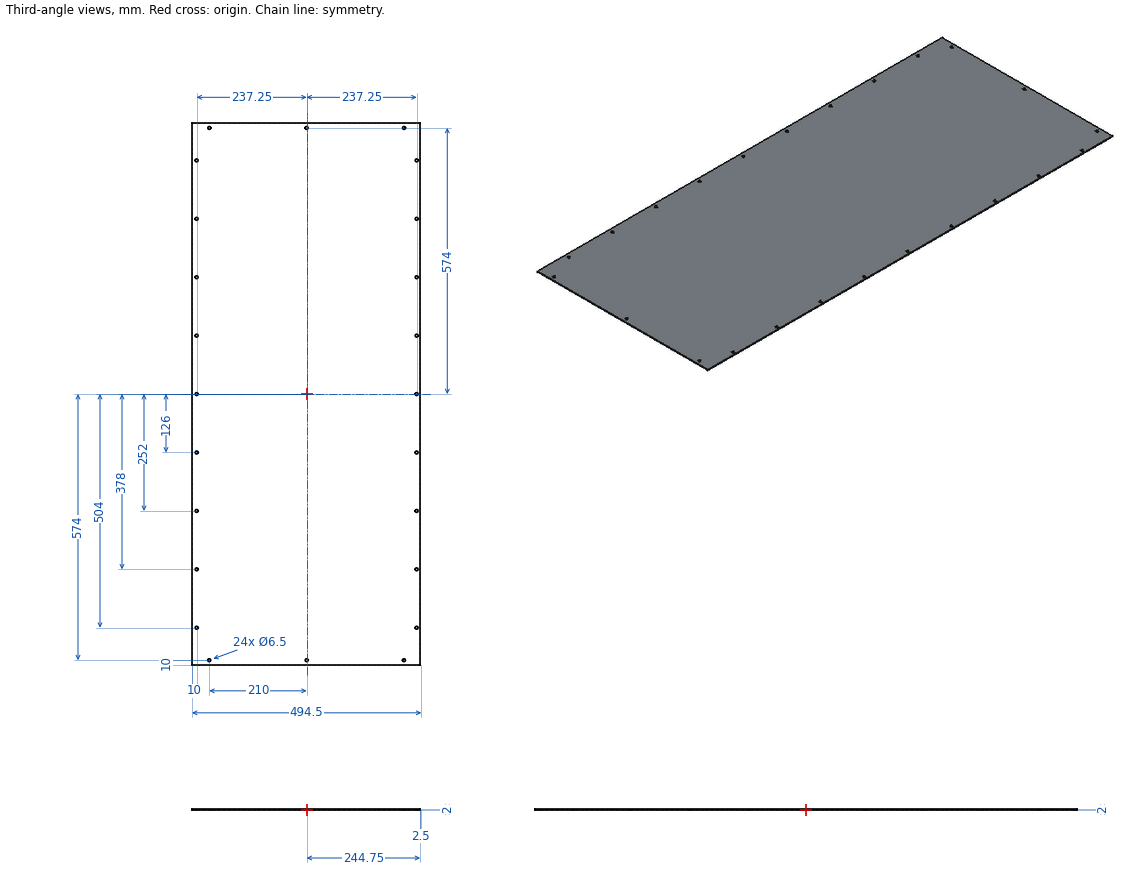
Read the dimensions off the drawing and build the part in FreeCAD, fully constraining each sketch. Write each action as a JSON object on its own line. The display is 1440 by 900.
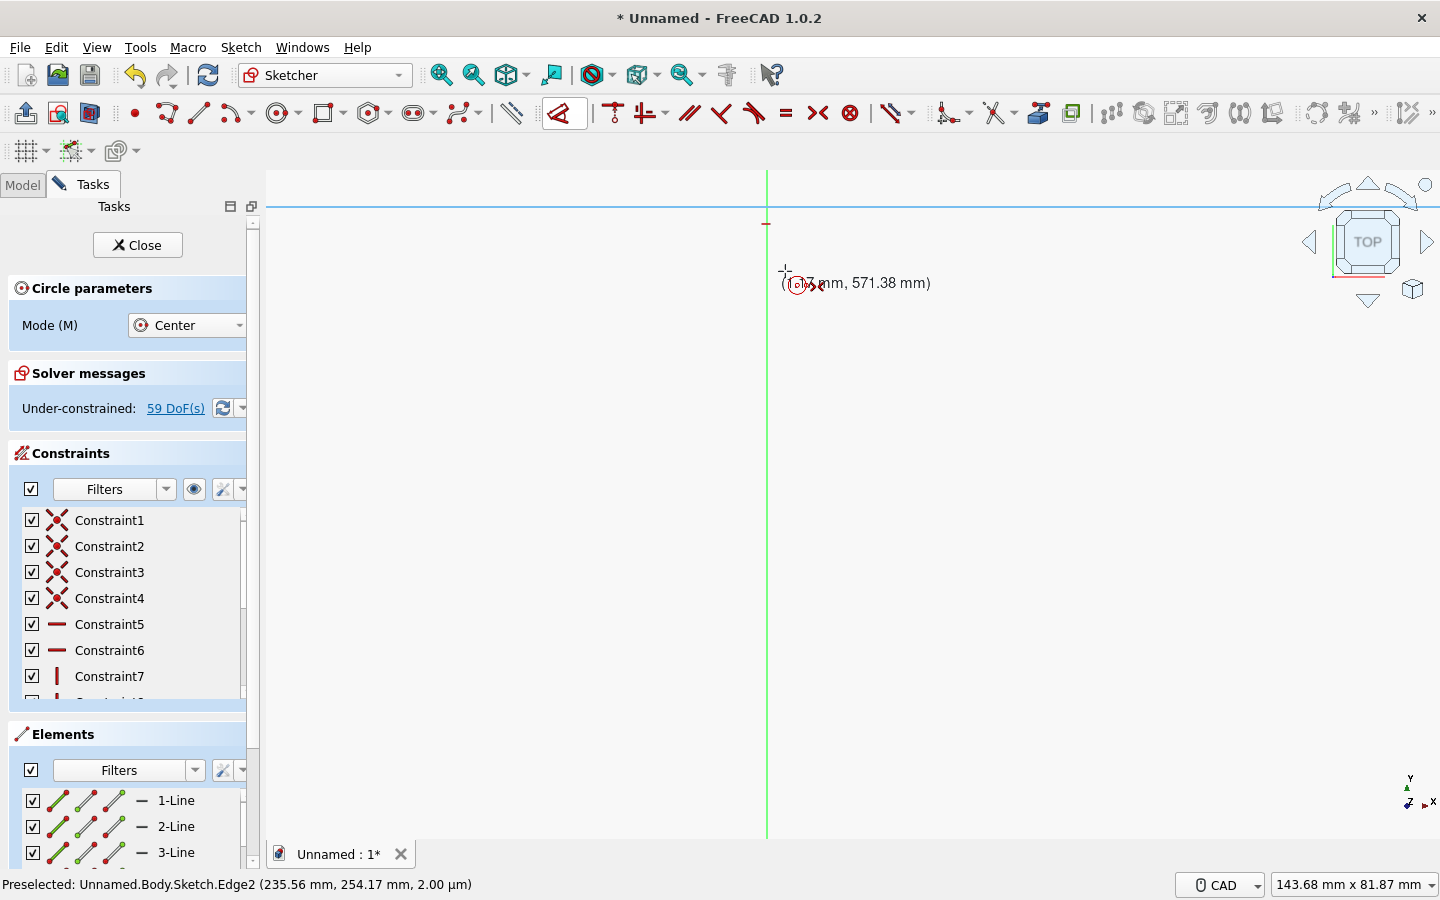
{"action": "scroll", "coordinate": [785, 271], "scroll_direction": "down", "scroll_amount": 15}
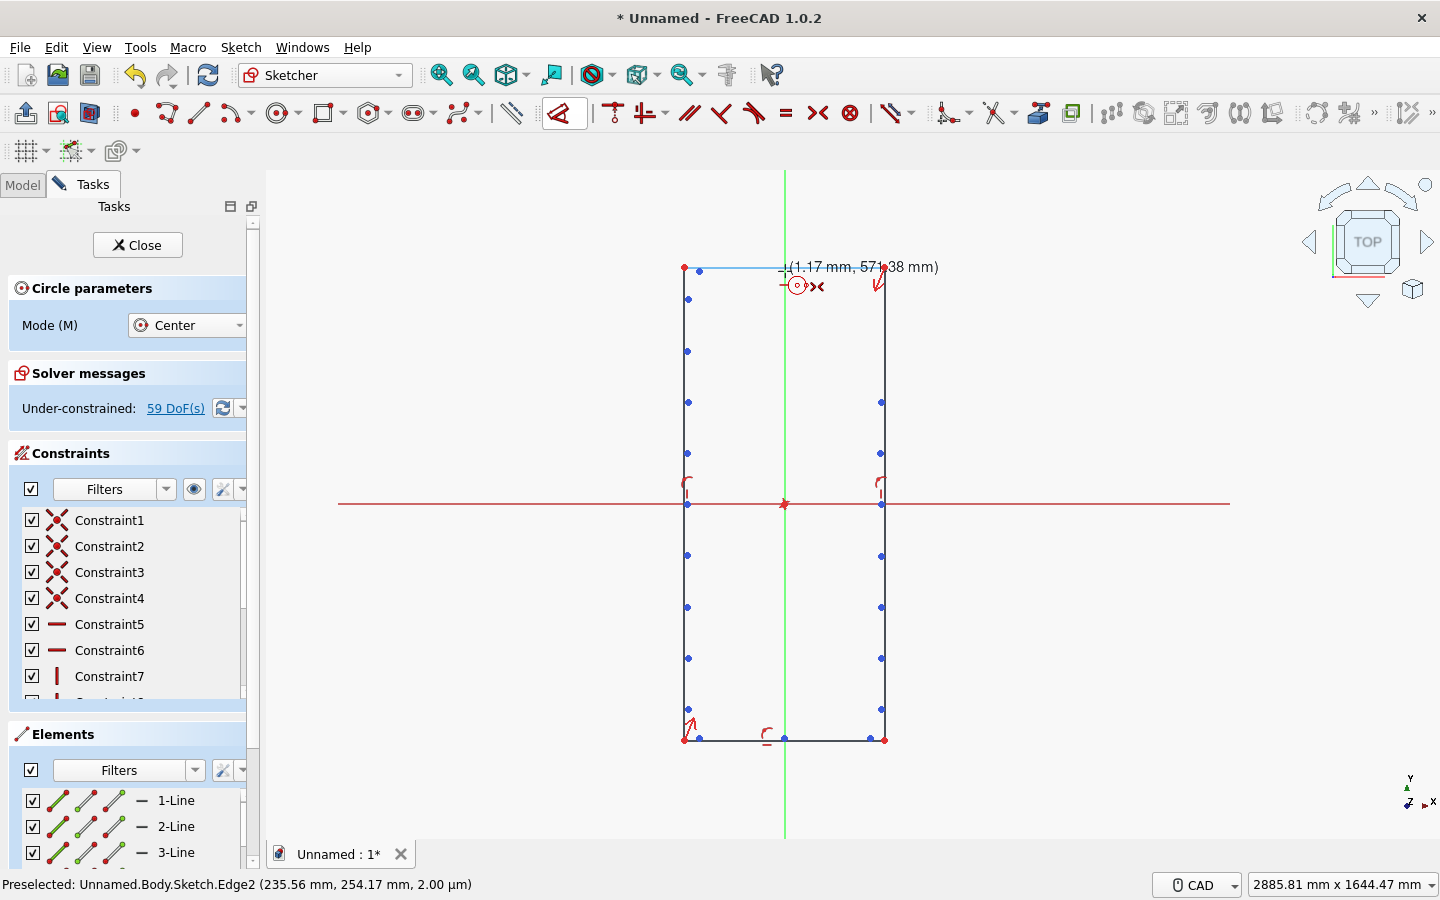
{"action": "scroll", "coordinate": [785, 271], "scroll_direction": "up", "scroll_amount": 7}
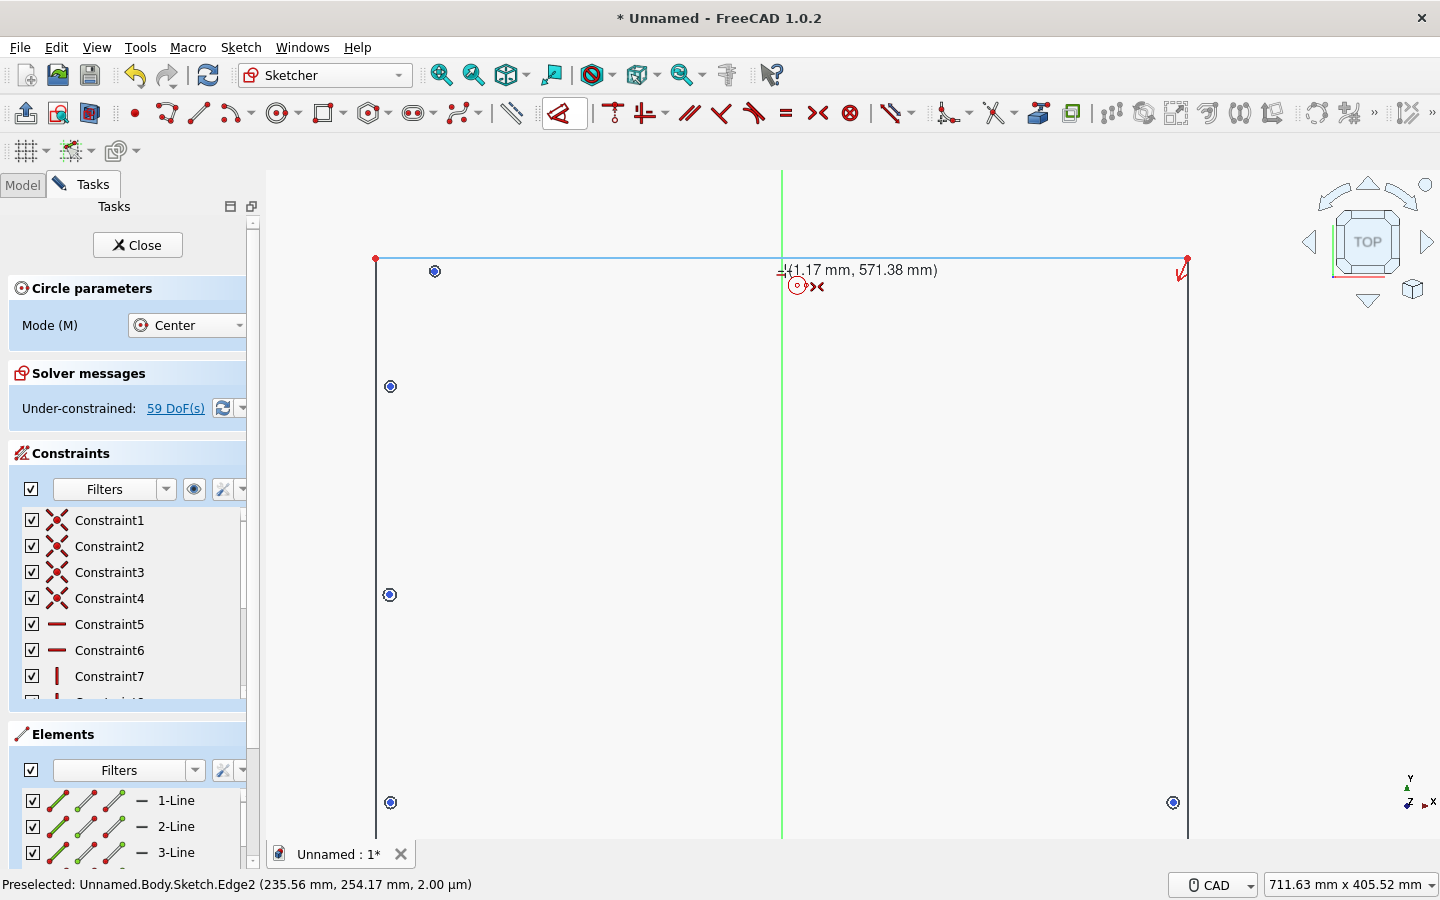
{"action": "left_click", "coordinate": [782, 270]}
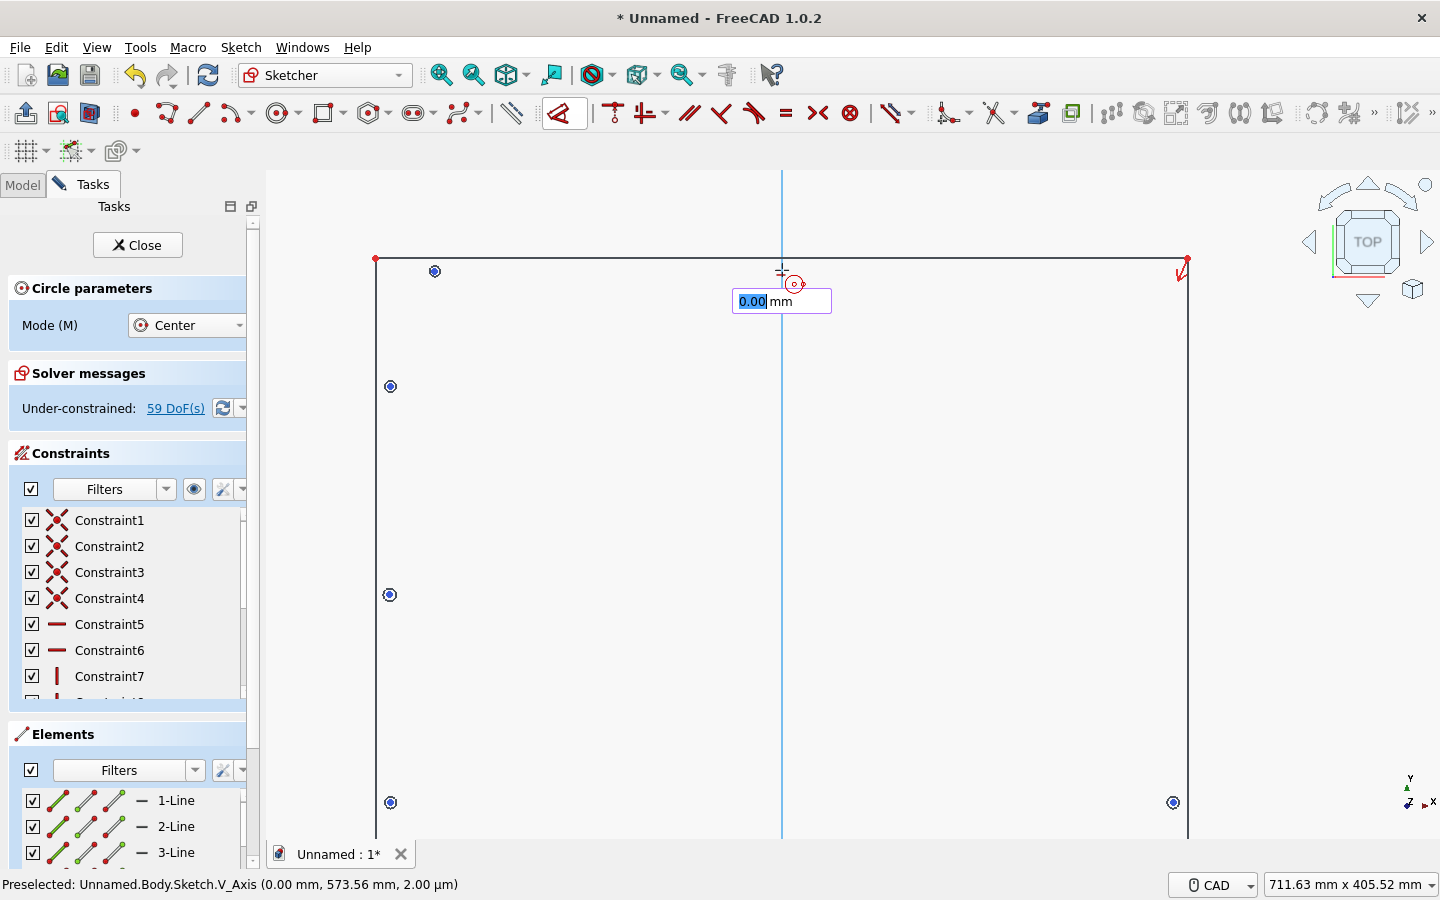
{"action": "scroll", "coordinate": [787, 268], "scroll_direction": "up", "scroll_amount": 6}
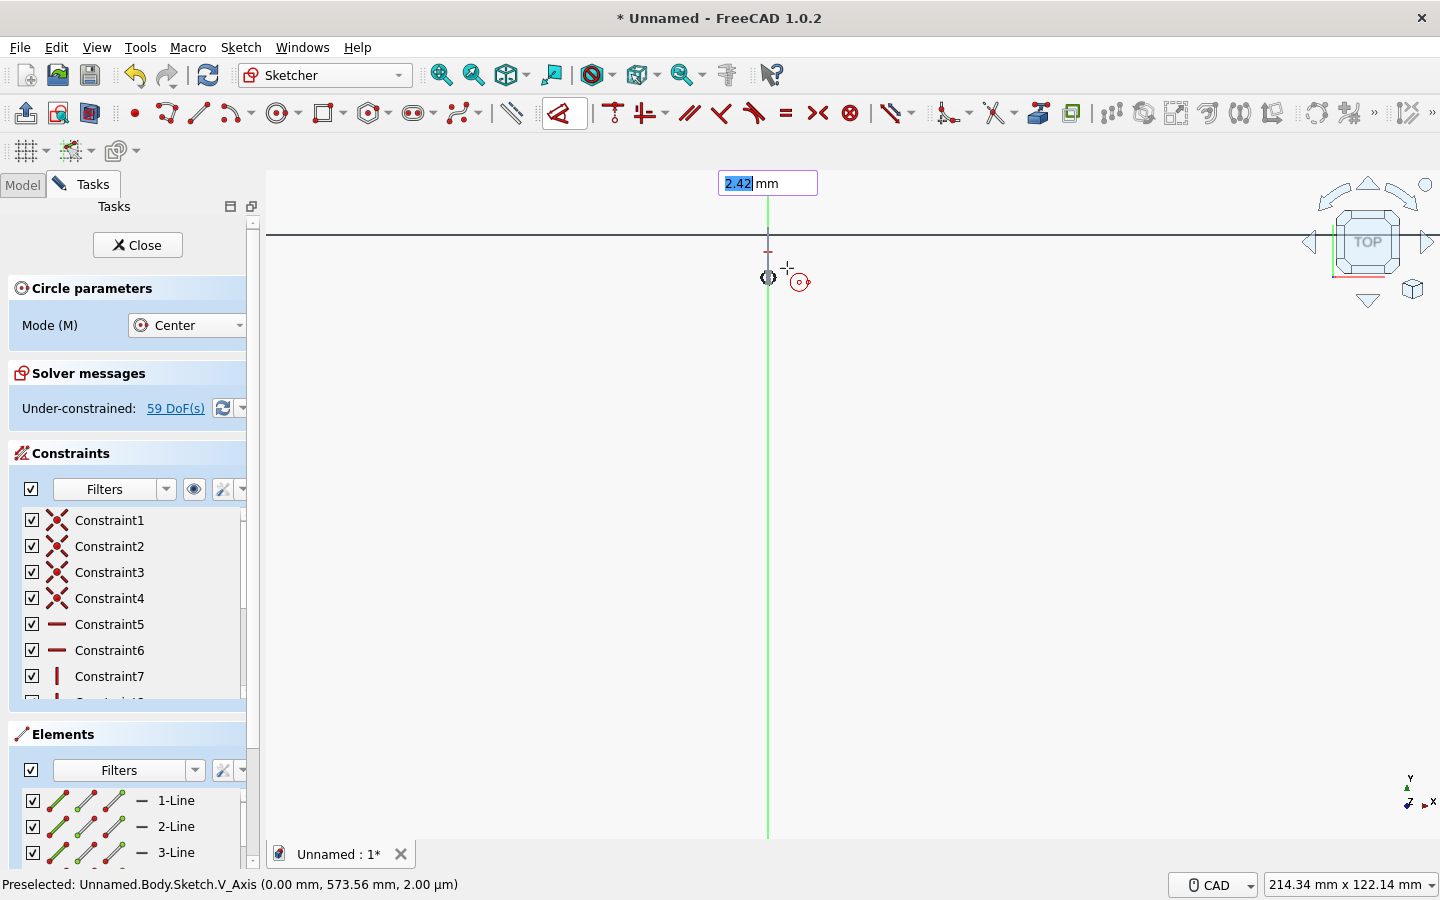
{"action": "left_click", "coordinate": [785, 269]}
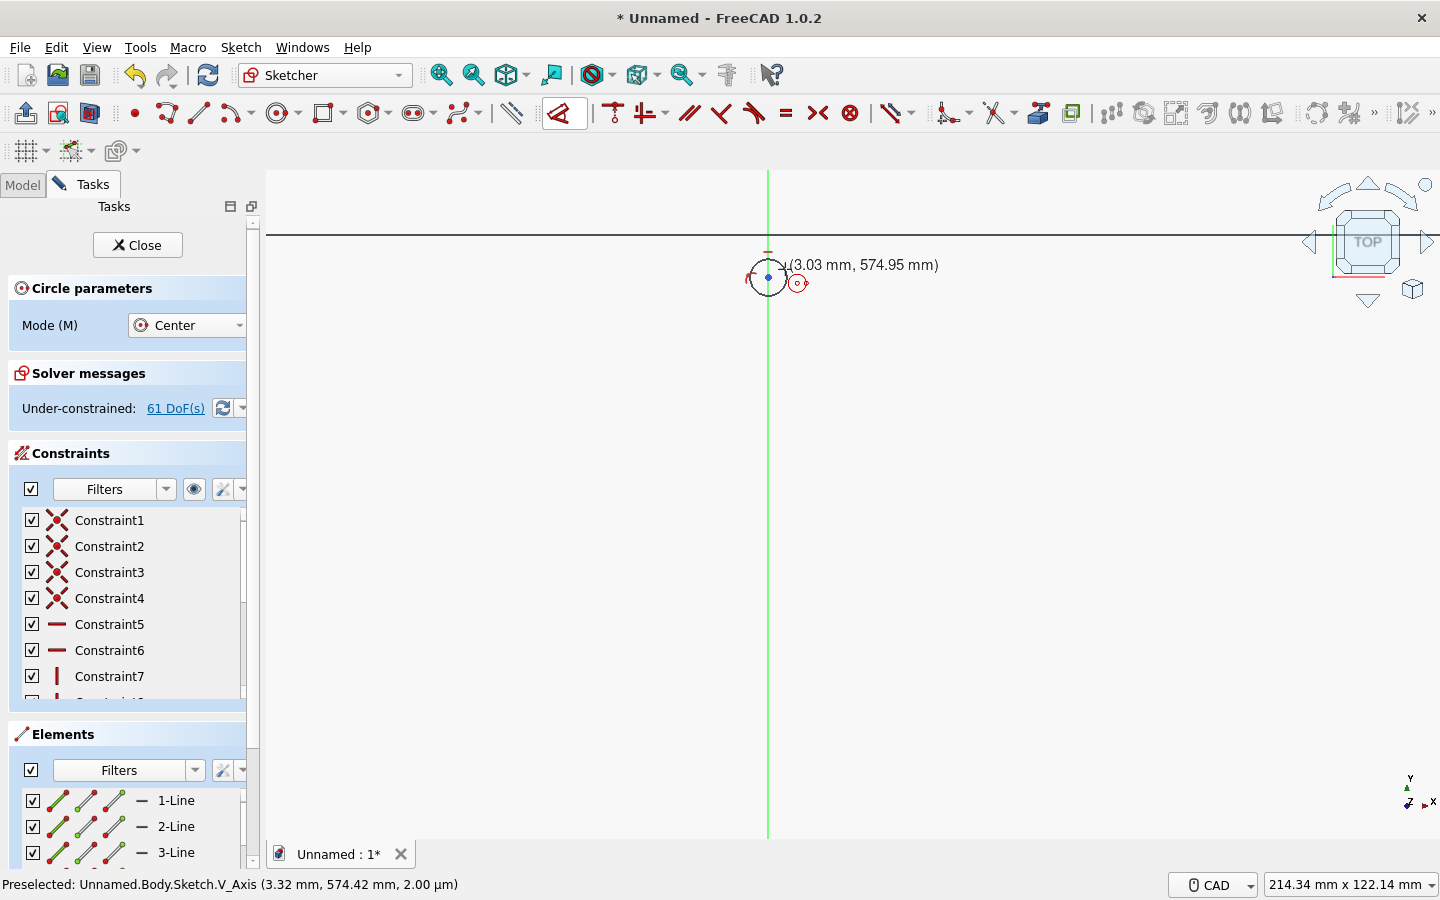
{"action": "scroll", "coordinate": [786, 271], "scroll_direction": "down", "scroll_amount": 13}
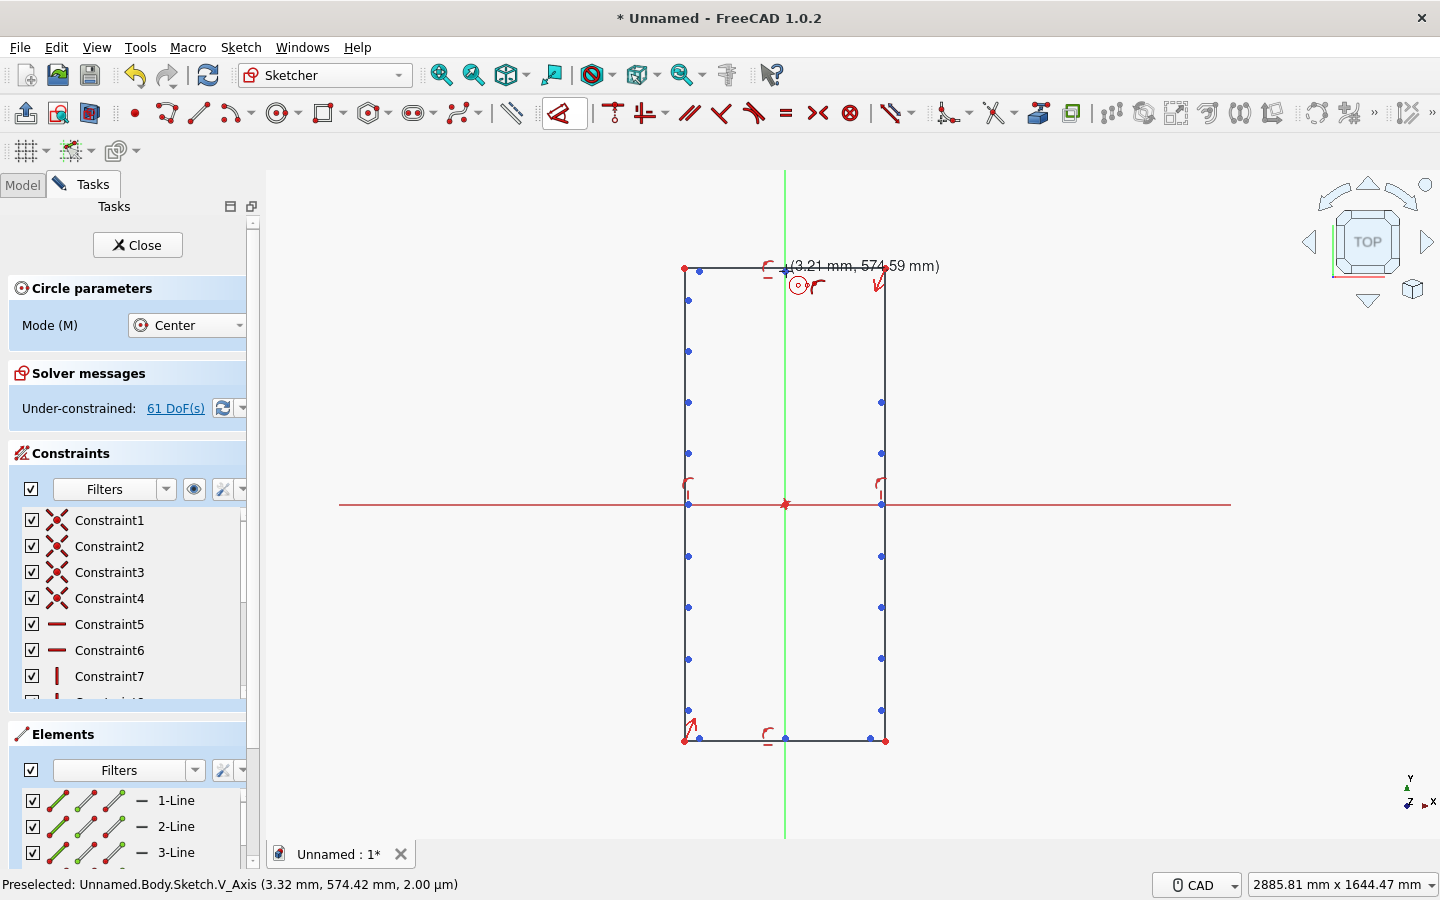
{"action": "scroll", "coordinate": [882, 351], "scroll_direction": "up", "scroll_amount": 15}